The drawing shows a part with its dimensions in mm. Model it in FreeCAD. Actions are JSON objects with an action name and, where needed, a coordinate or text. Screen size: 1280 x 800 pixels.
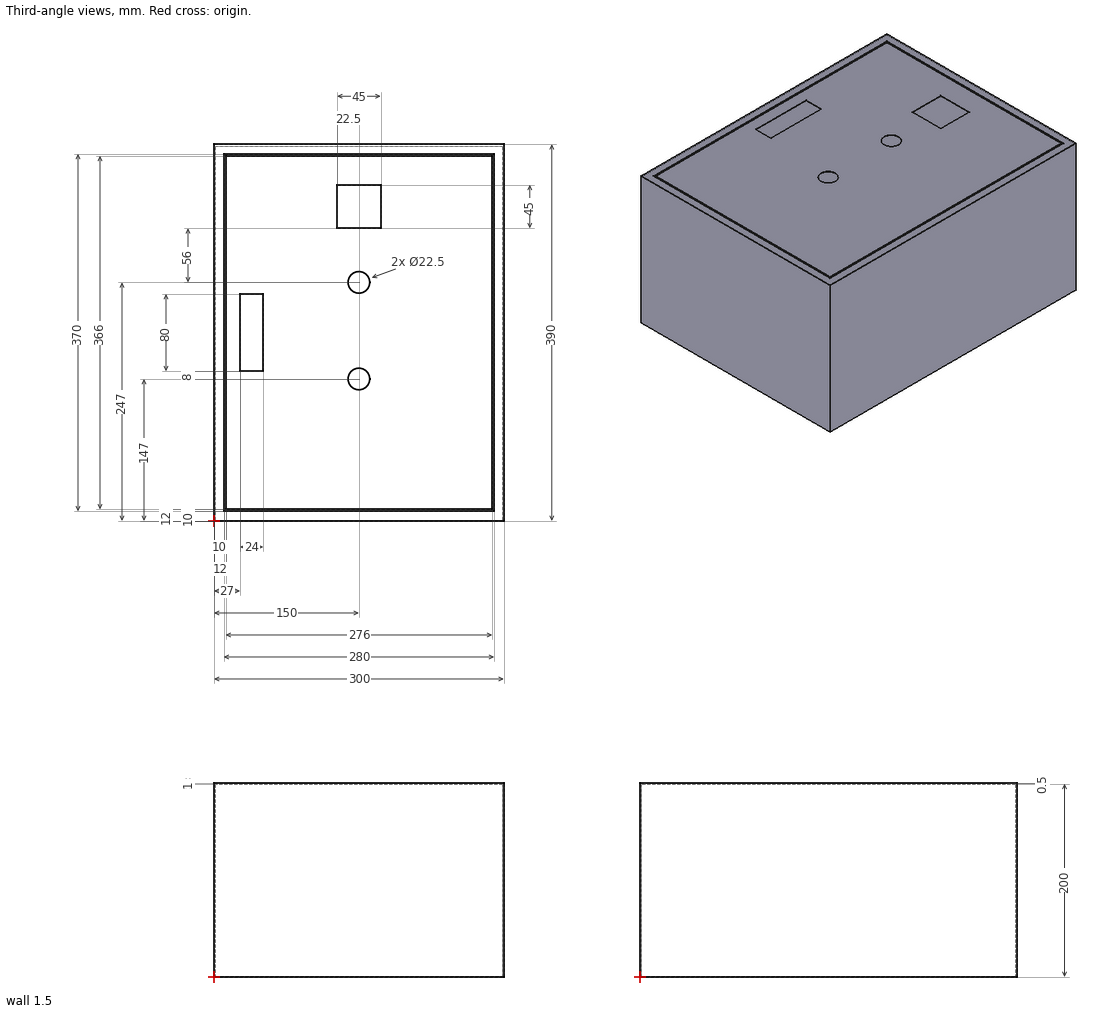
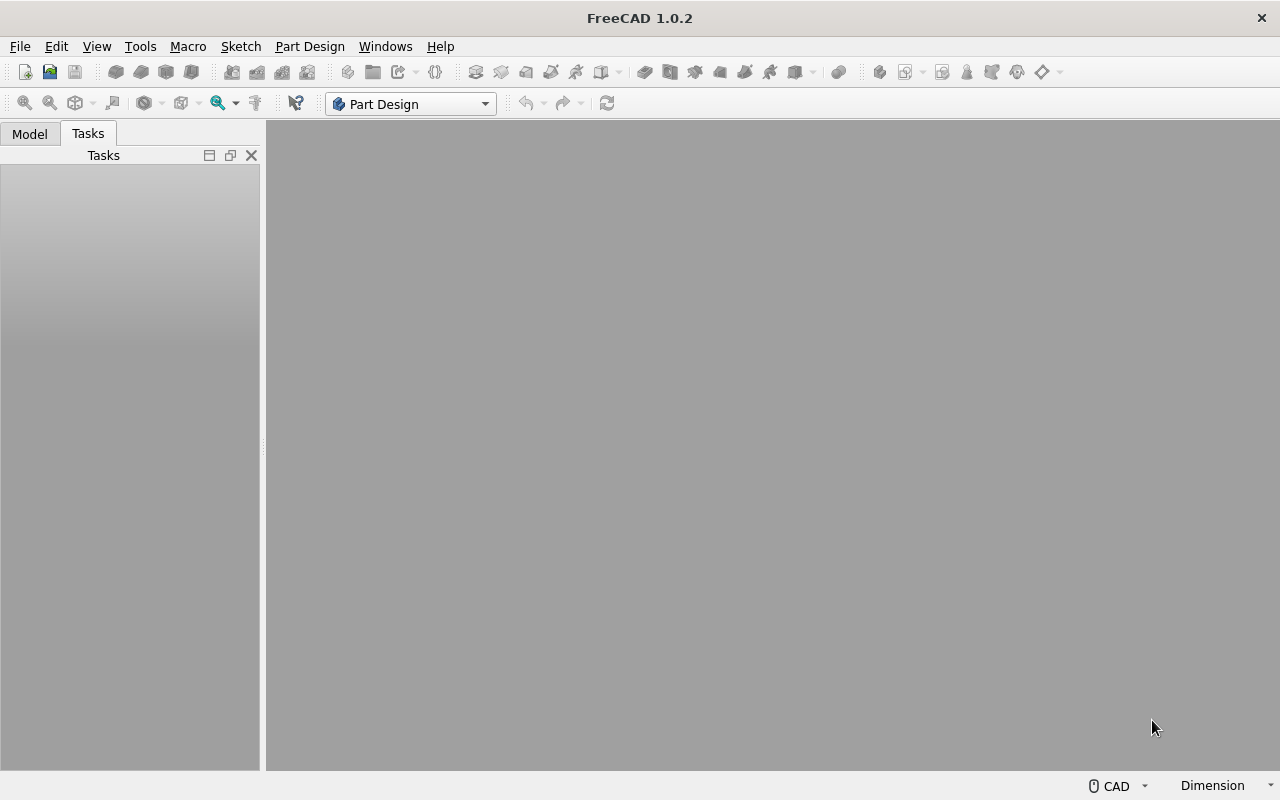
{"action": "left_click", "coordinate": [25, 72]}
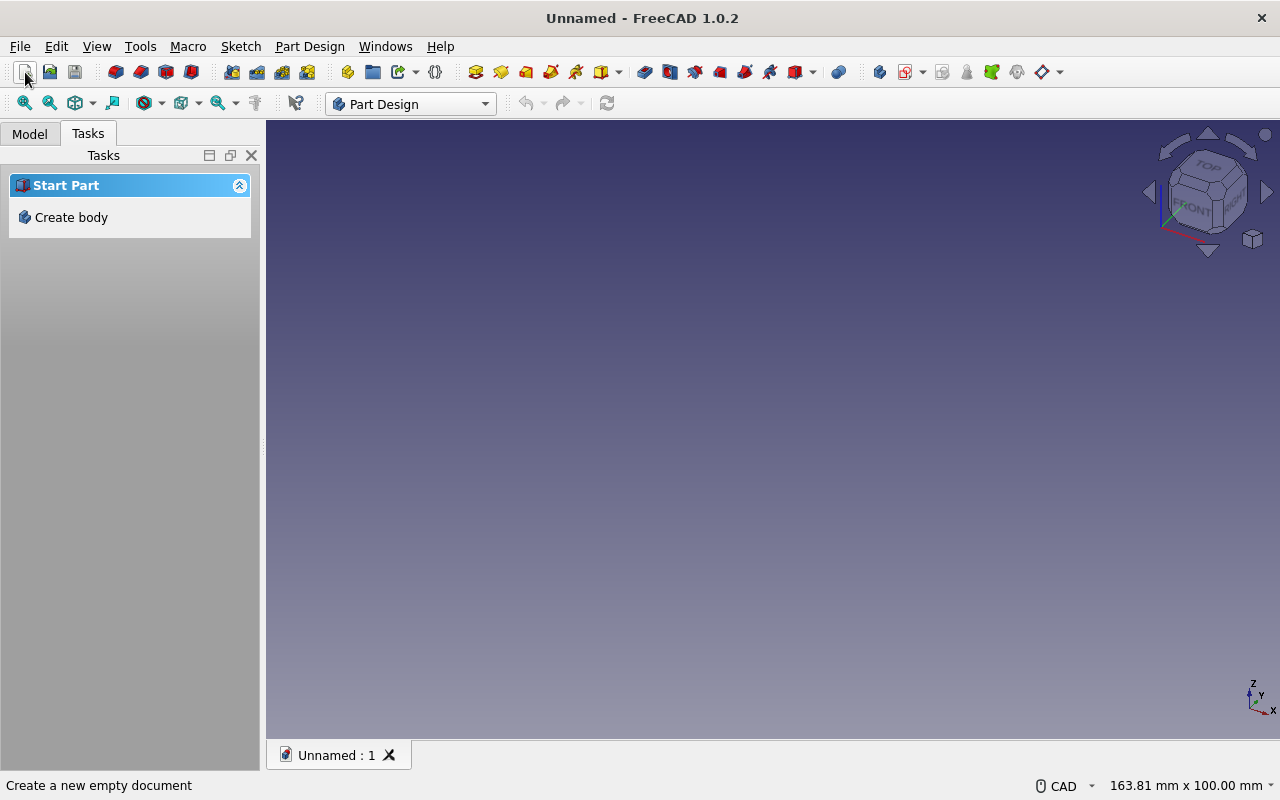
{"action": "left_click", "coordinate": [904, 72]}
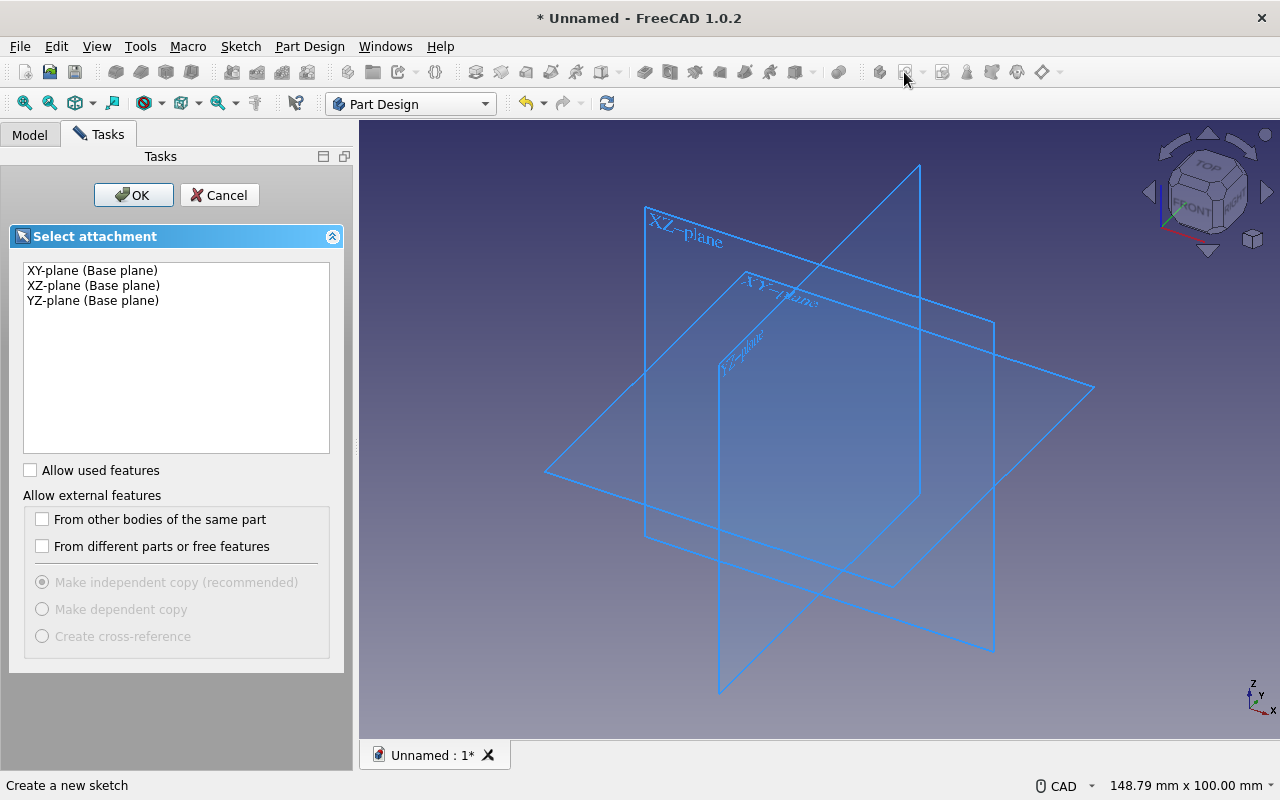
{"action": "left_click", "coordinate": [84, 270]}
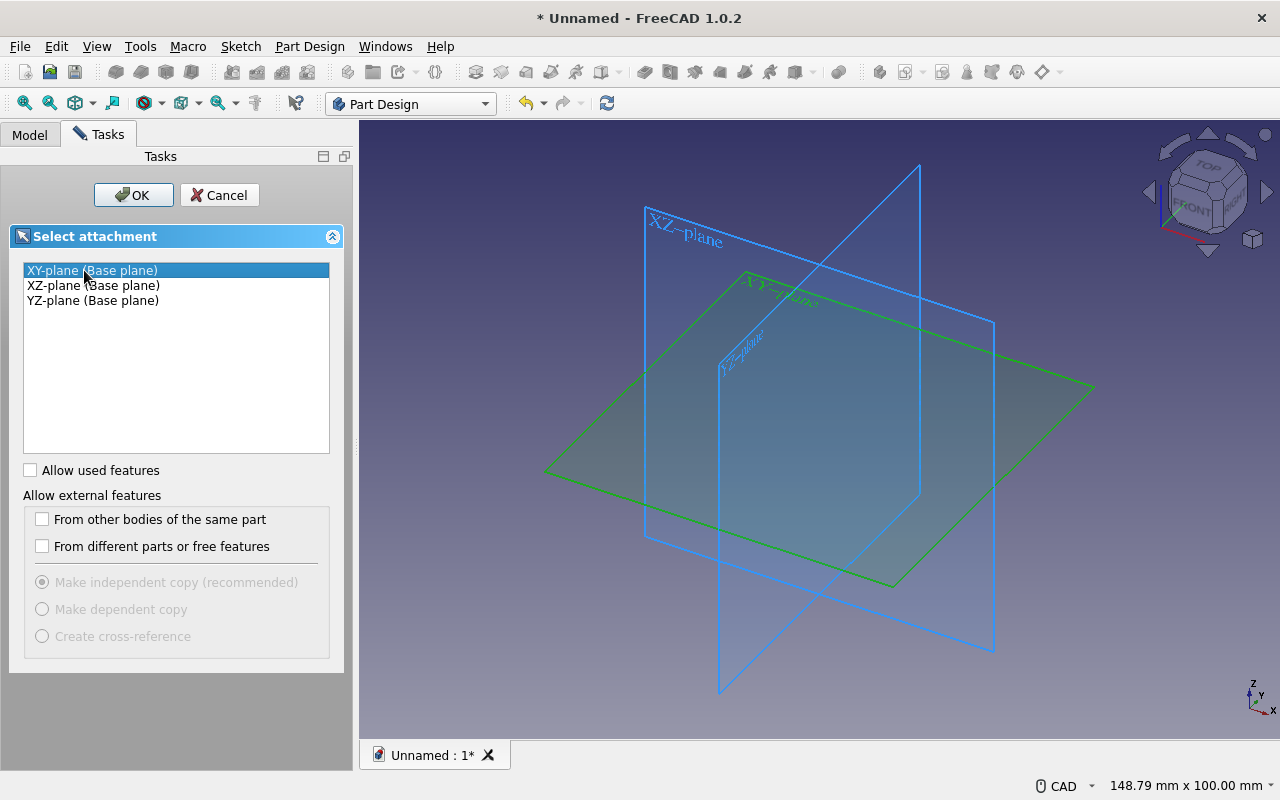
{"action": "left_click", "coordinate": [134, 195]}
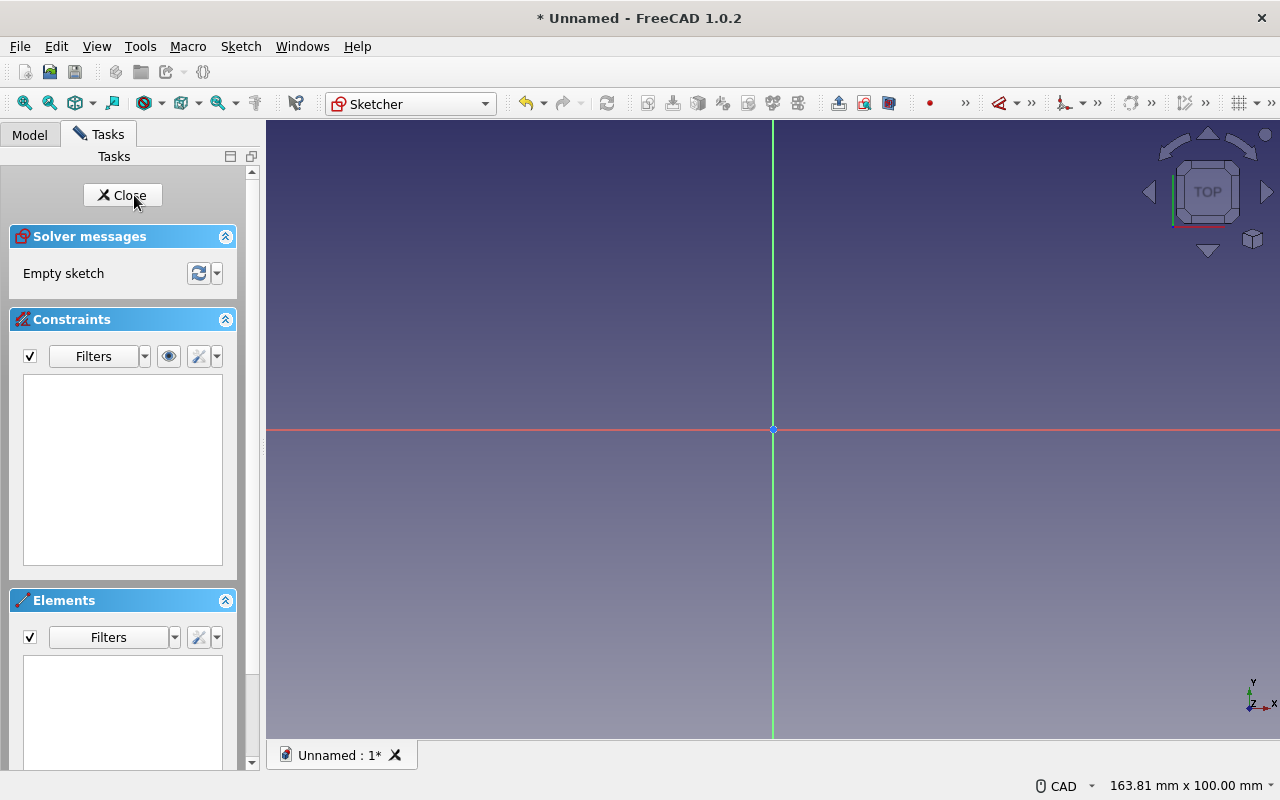
{"action": "scroll", "coordinate": [507, 669], "scroll_direction": "down", "scroll_amount": 9}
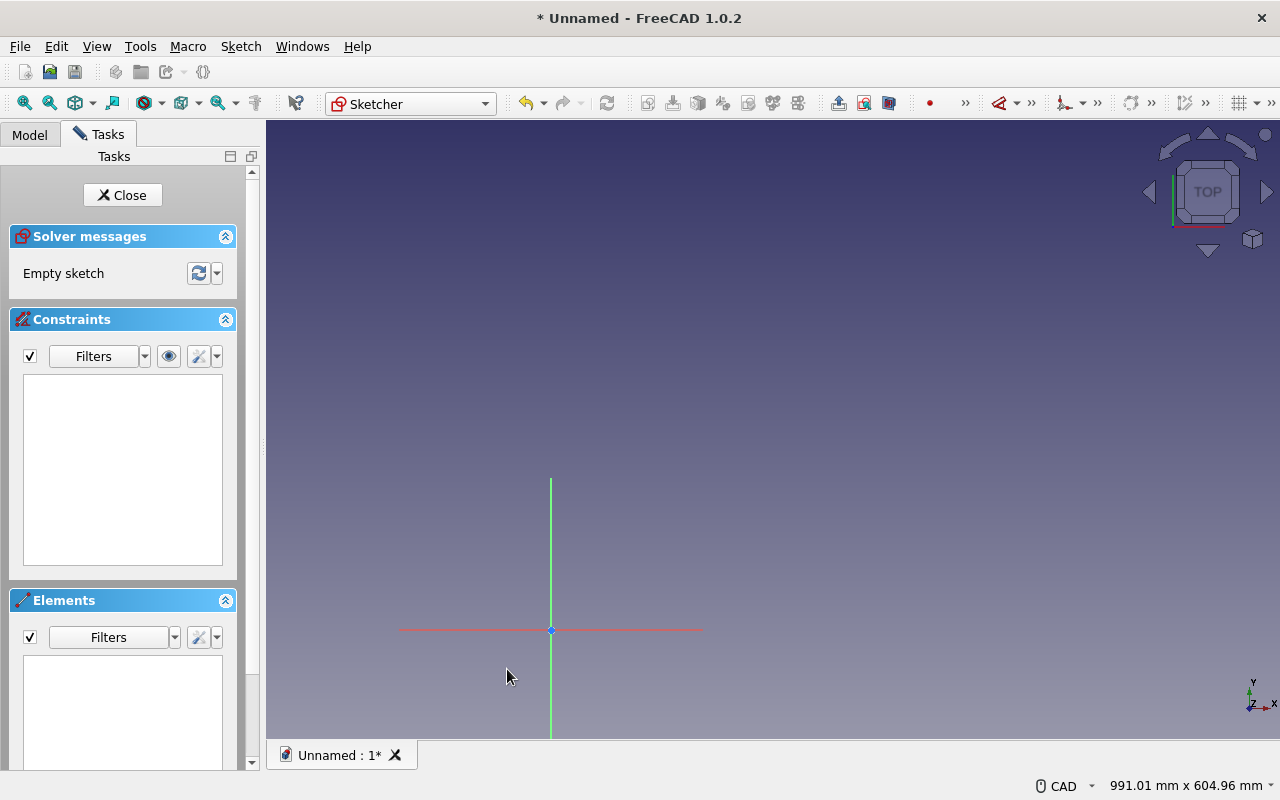
{"action": "key", "text": "g r"}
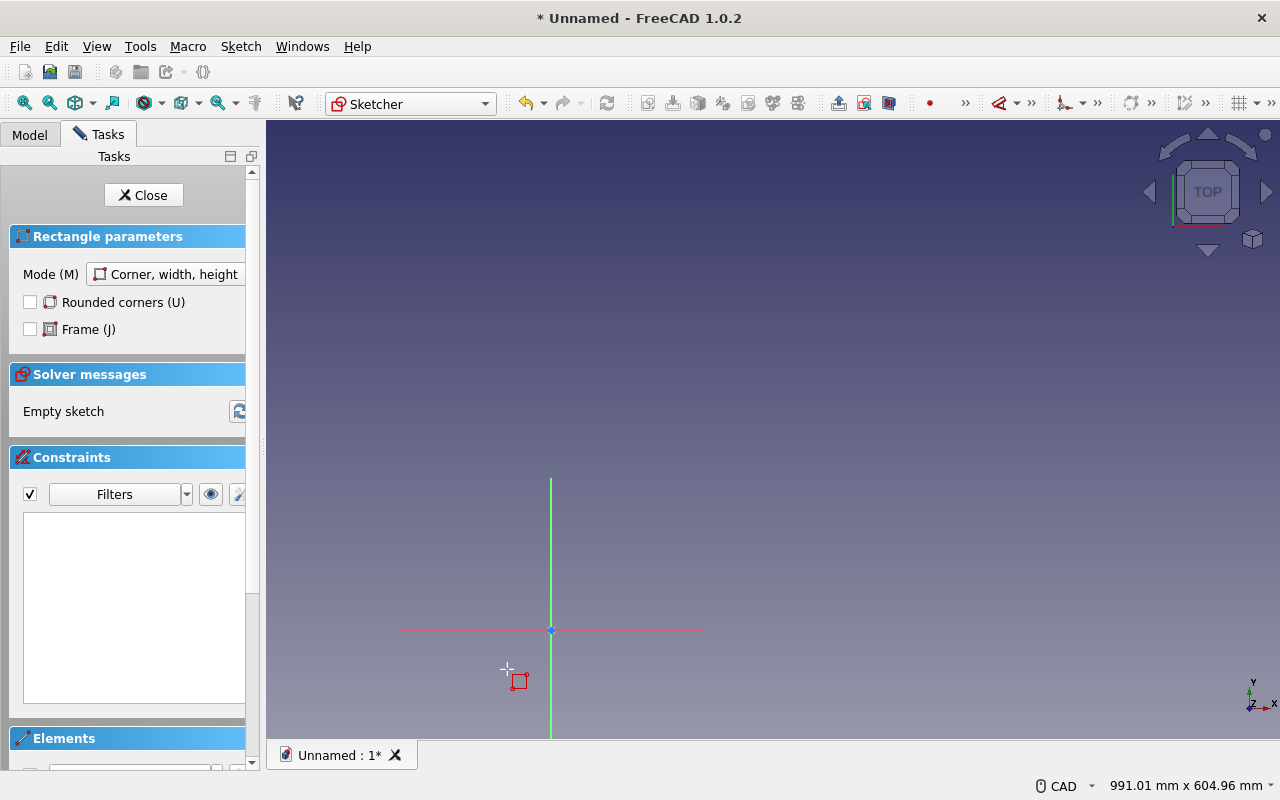
{"action": "left_click", "coordinate": [551, 630]}
{"action": "mouse_move", "coordinate": [858, 231]}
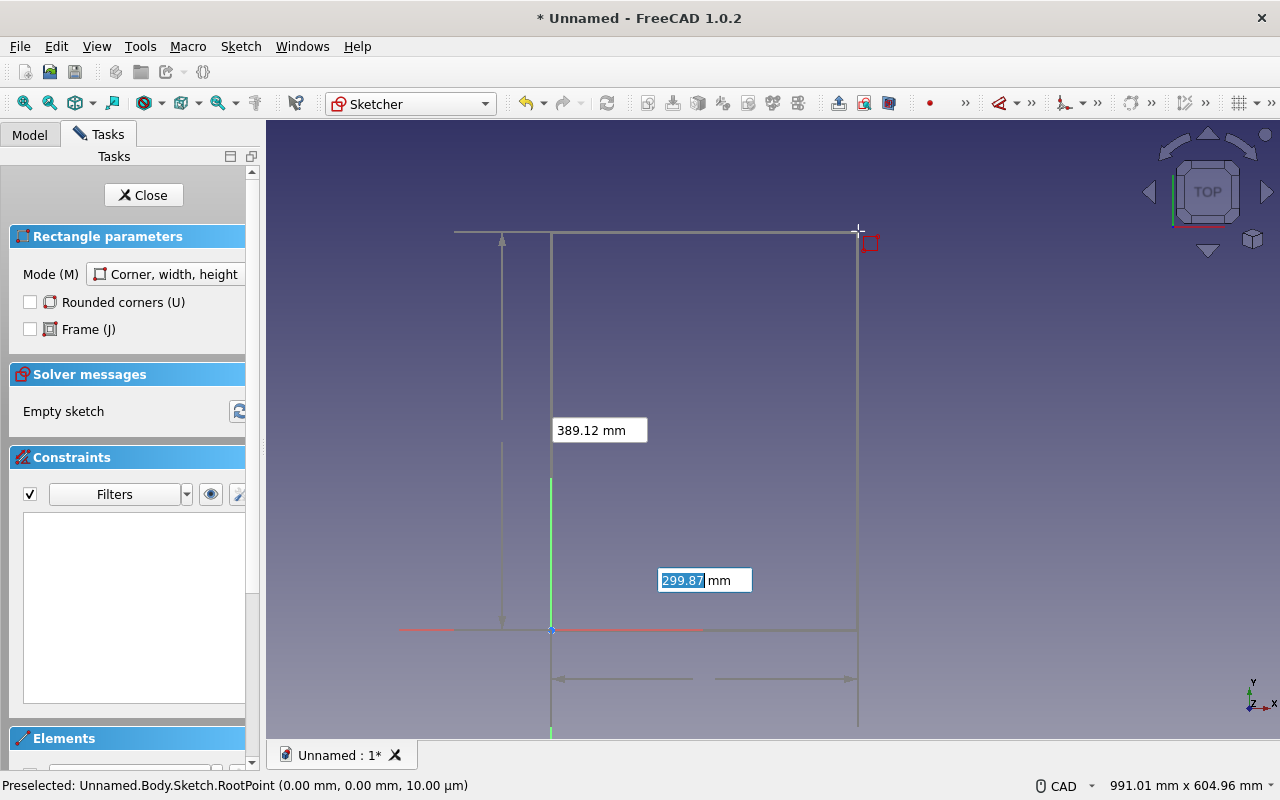
{"action": "type", "text": "300"}
{"action": "key", "text": "Tab"}
{"action": "type", "text": "390"}
{"action": "key", "text": "Return"}
{"action": "key", "text": "Escape"}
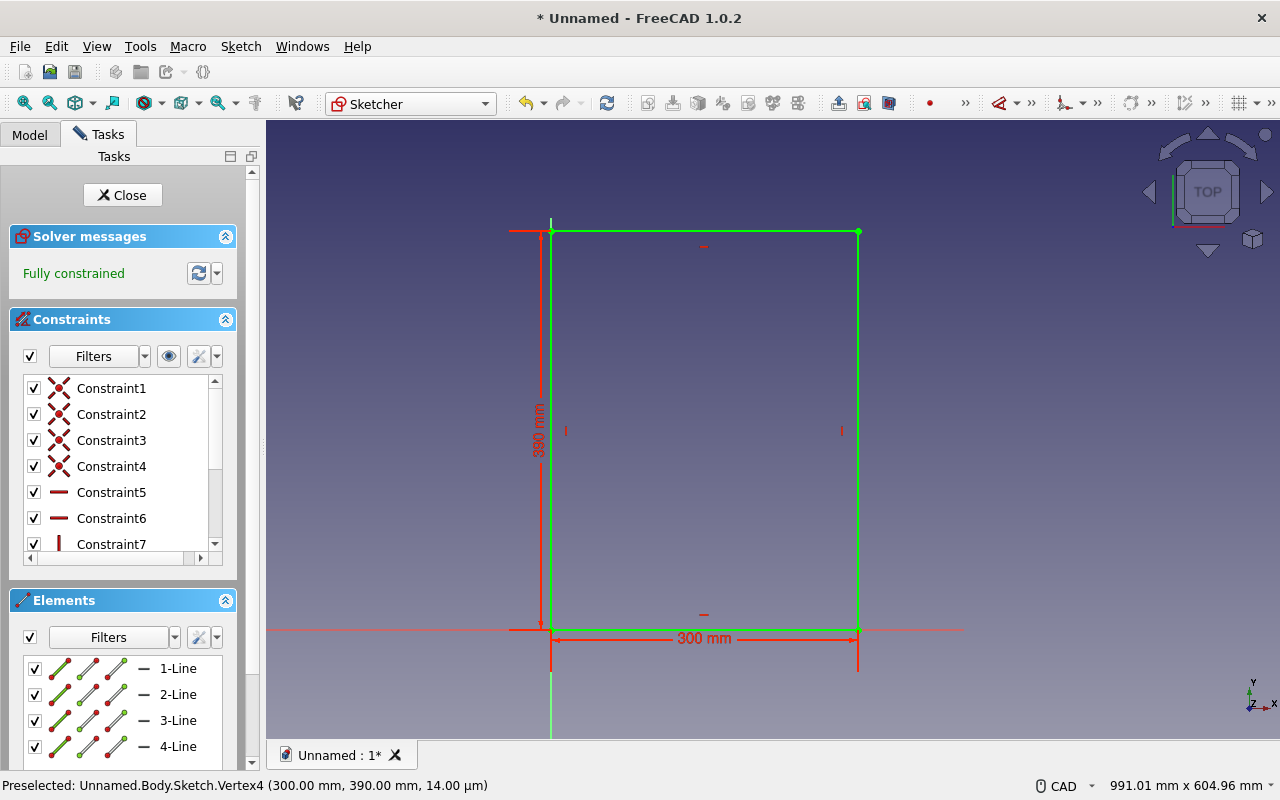
{"action": "left_click", "coordinate": [123, 195]}